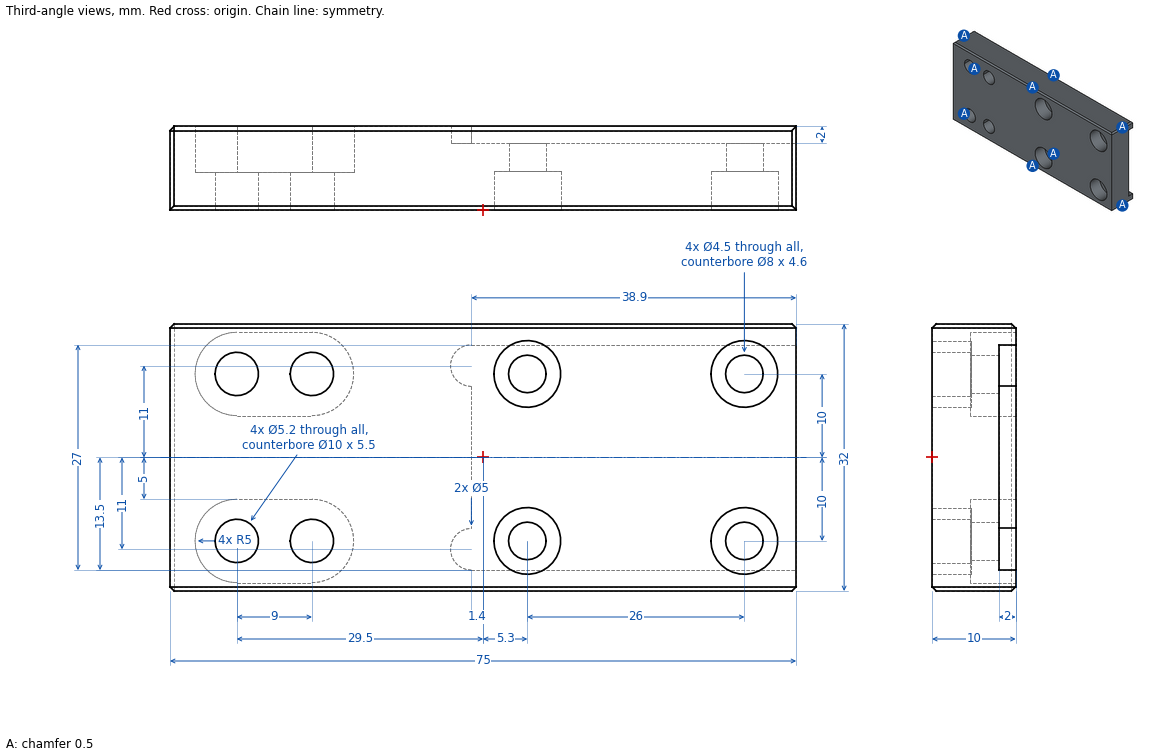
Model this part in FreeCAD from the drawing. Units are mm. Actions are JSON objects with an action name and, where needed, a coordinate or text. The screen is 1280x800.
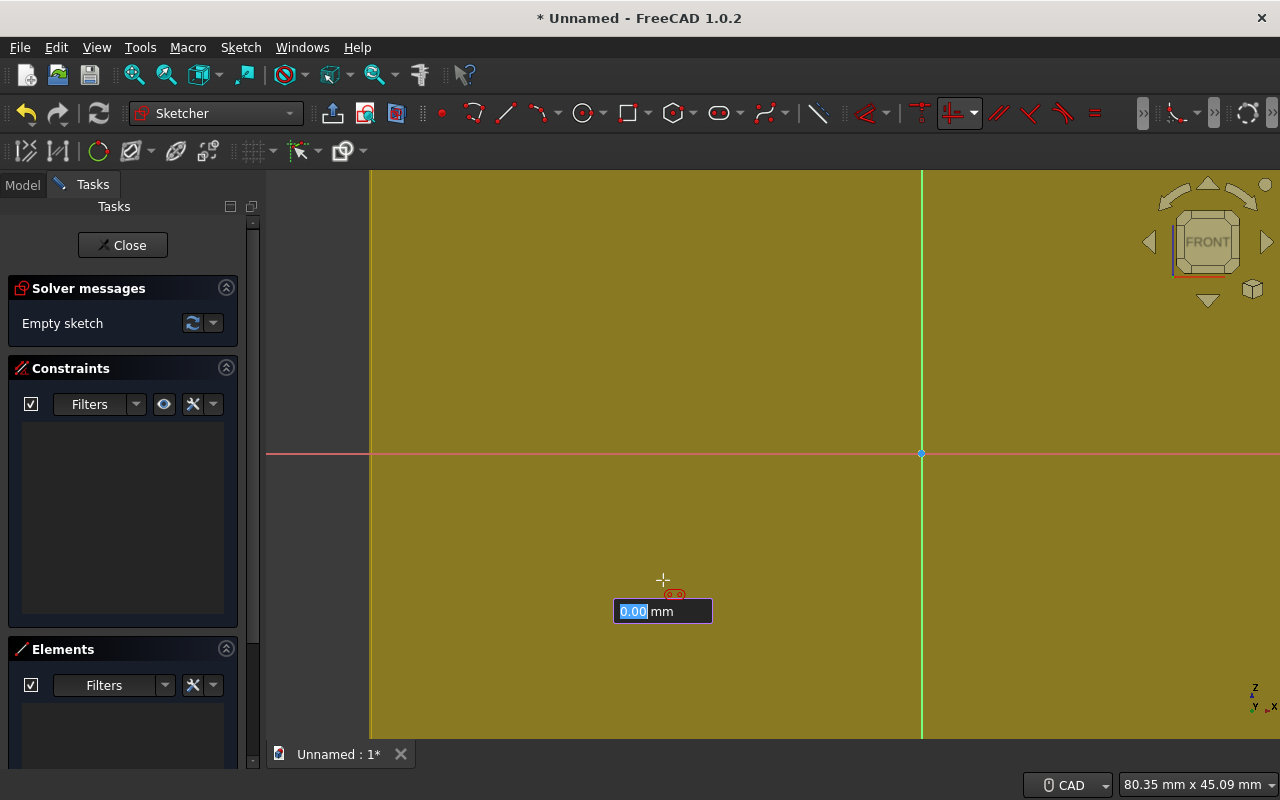
{"action": "left_click", "coordinate": [606, 643]}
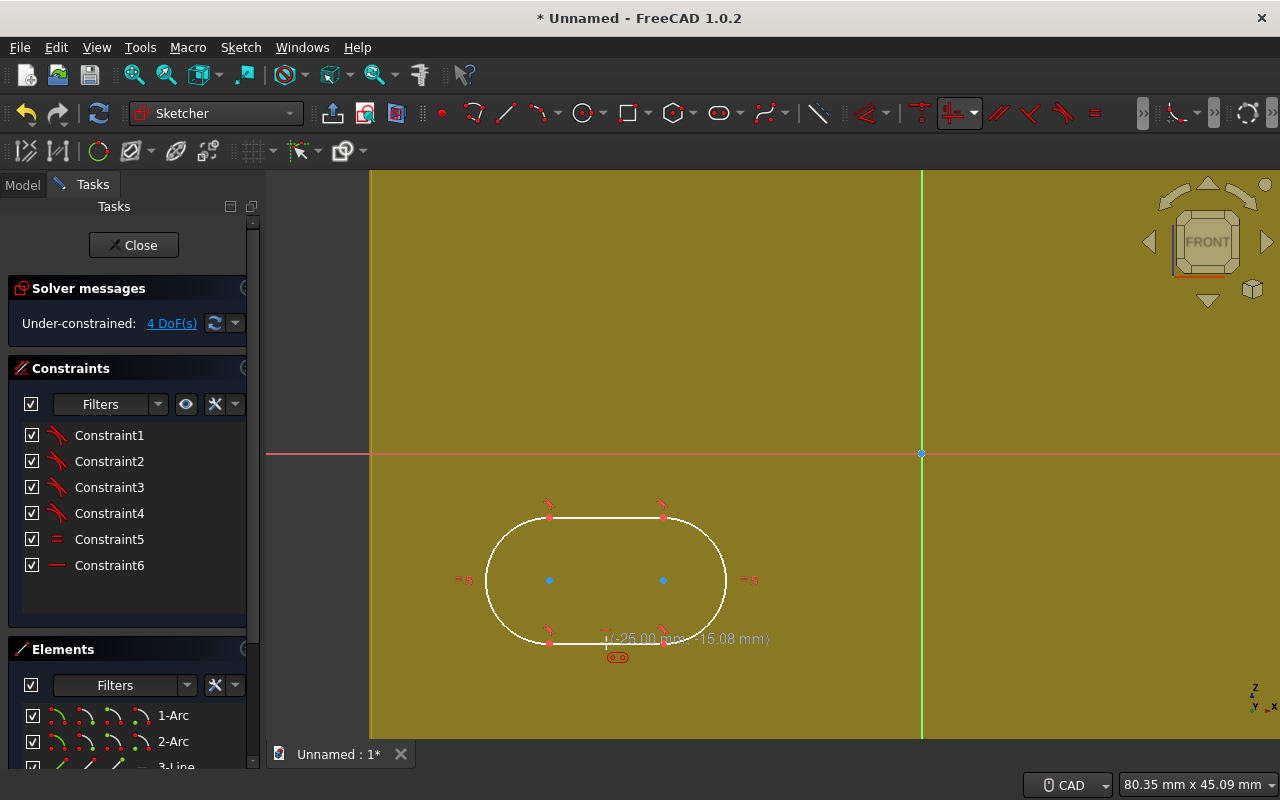
{"action": "left_click", "coordinate": [549, 327]}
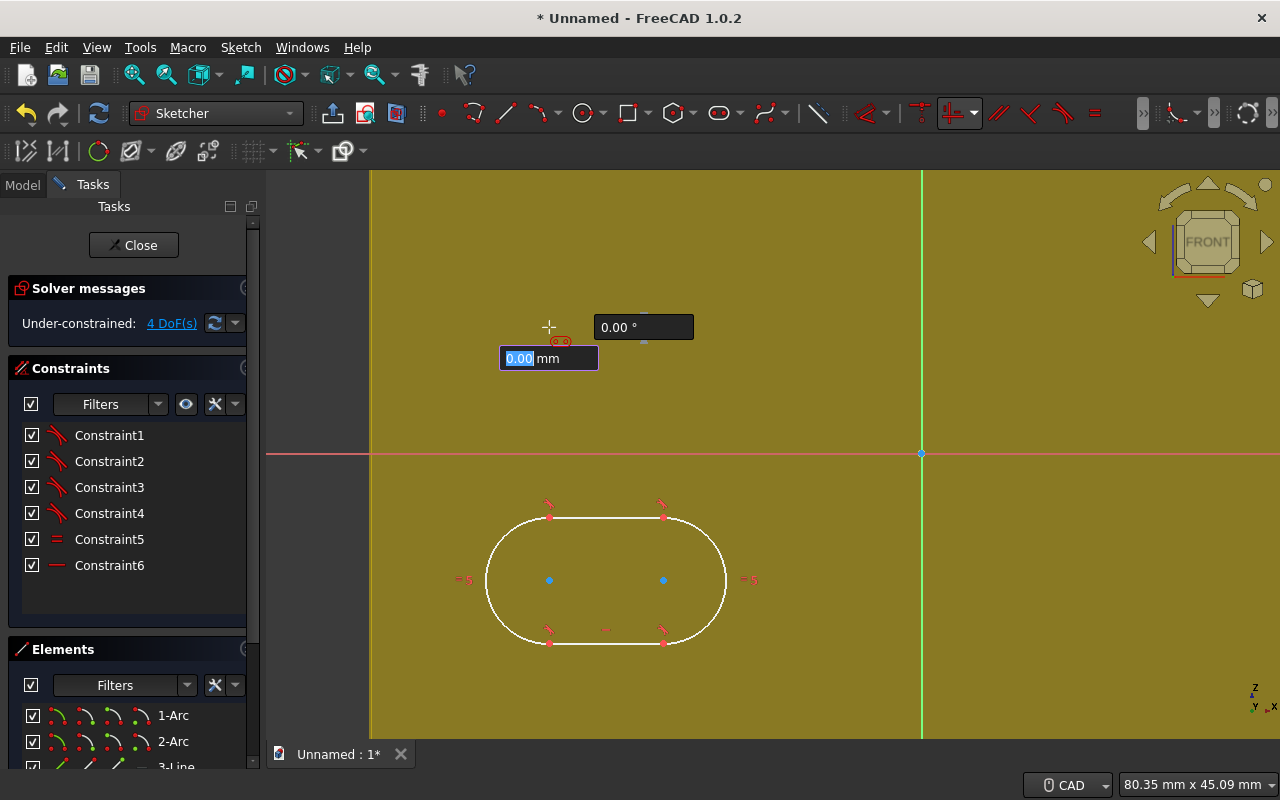
{"action": "left_click", "coordinate": [663, 327]}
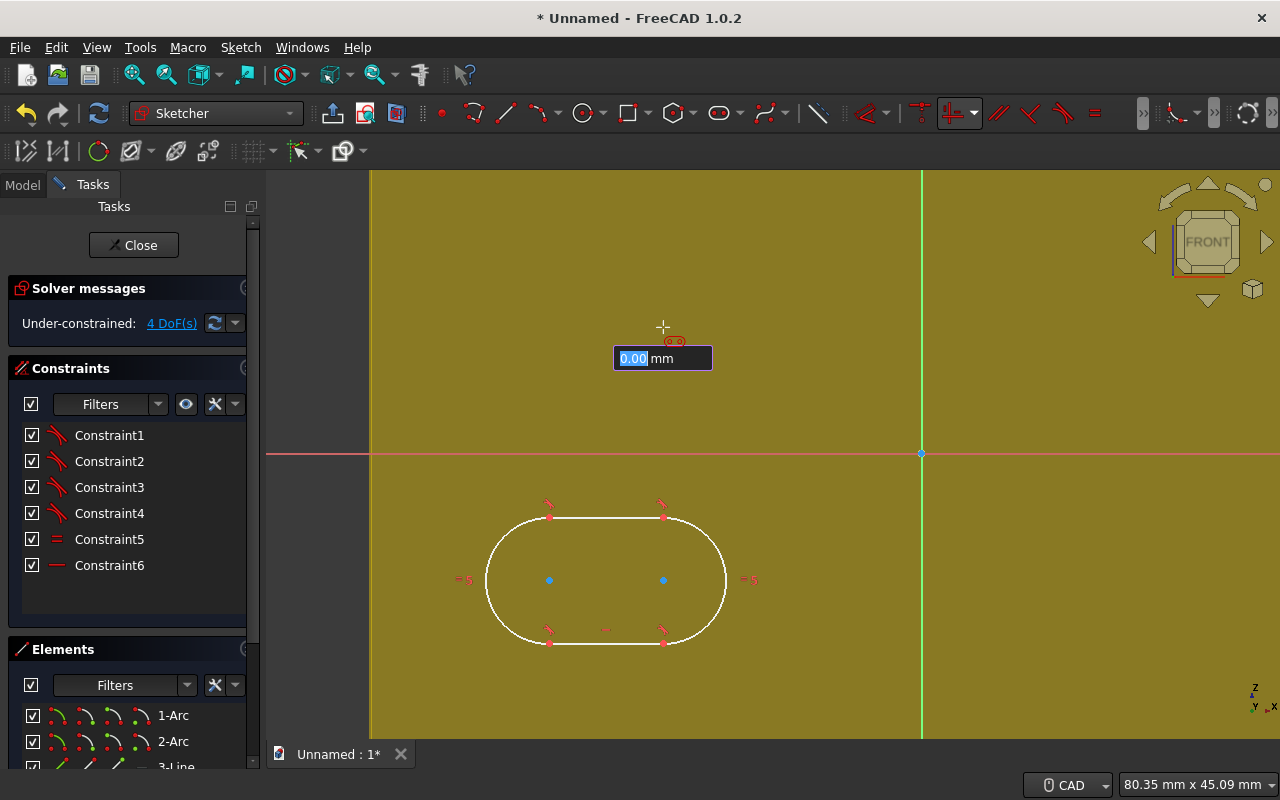
{"action": "left_click", "coordinate": [606, 391]}
{"action": "key", "text": "Escape"}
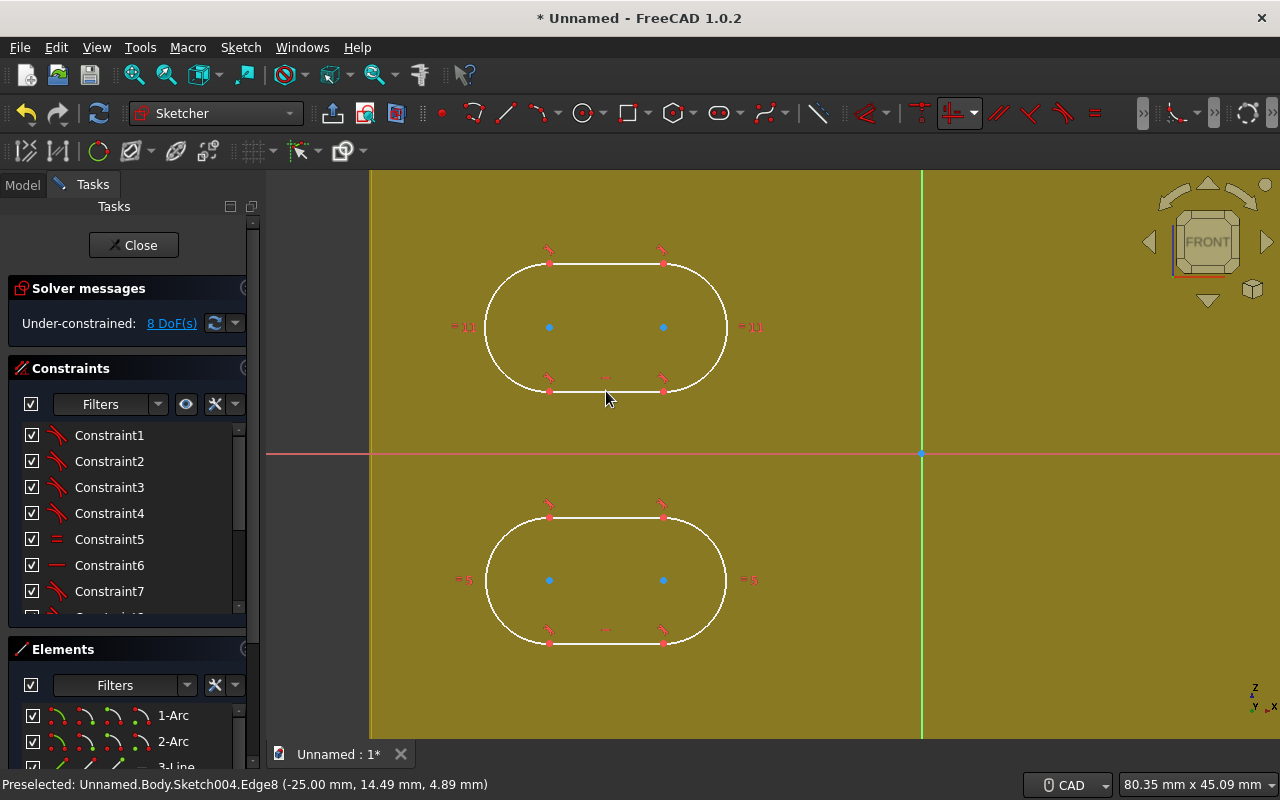
{"action": "left_click", "coordinate": [498, 544]}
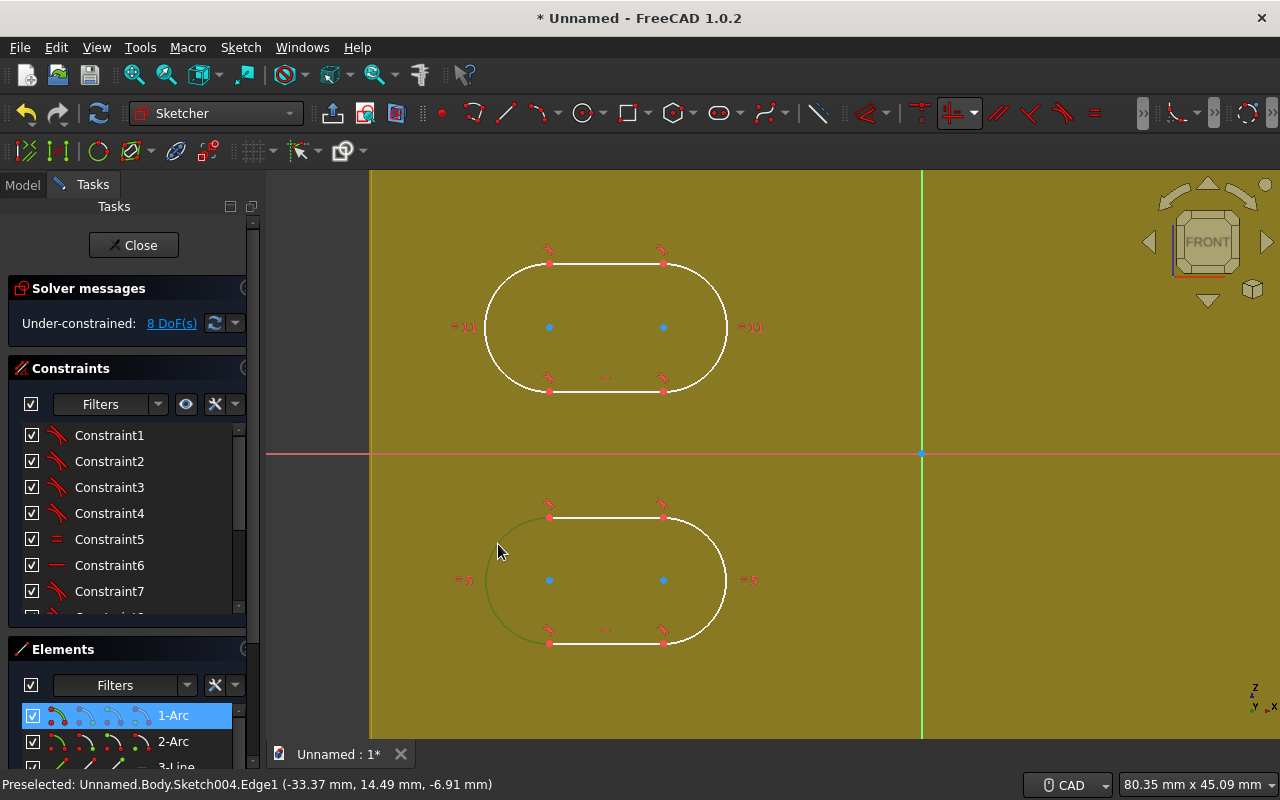
{"action": "left_click", "coordinate": [497, 290]}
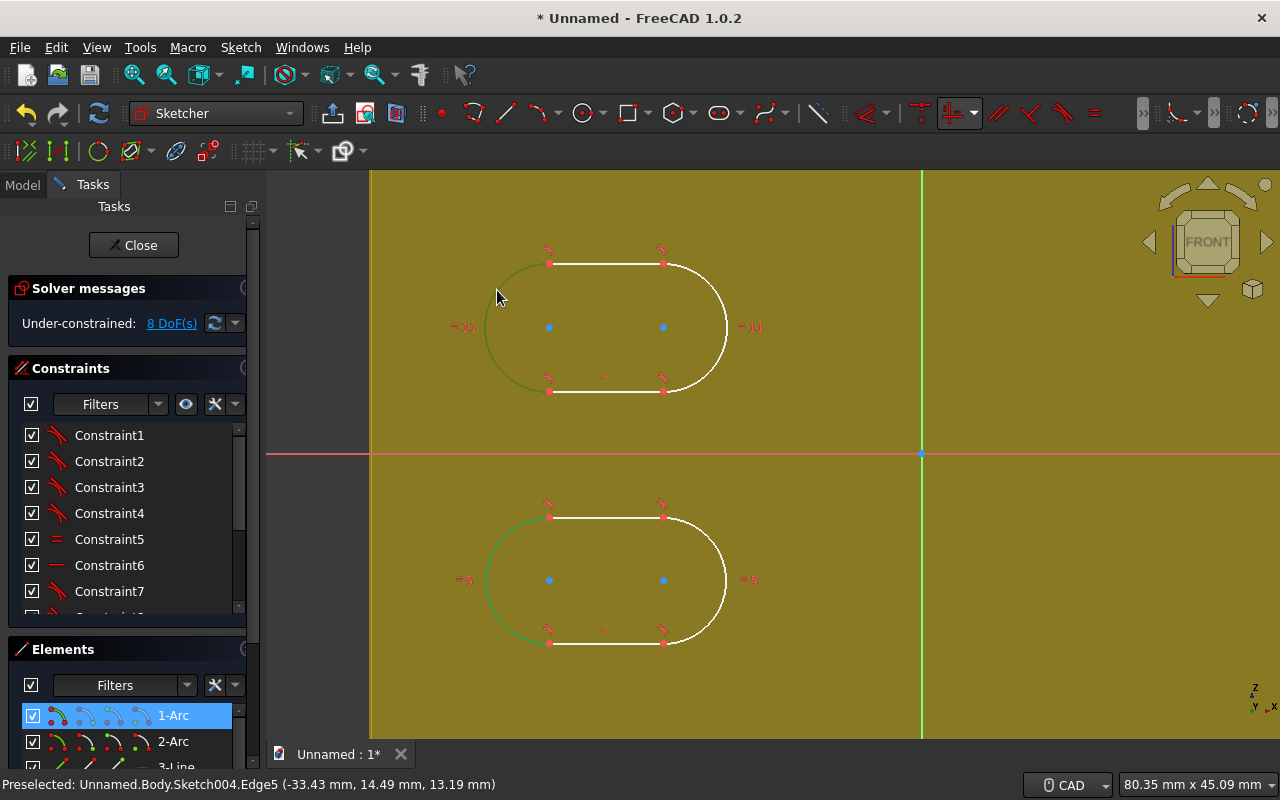
{"action": "left_click", "coordinate": [1096, 114]}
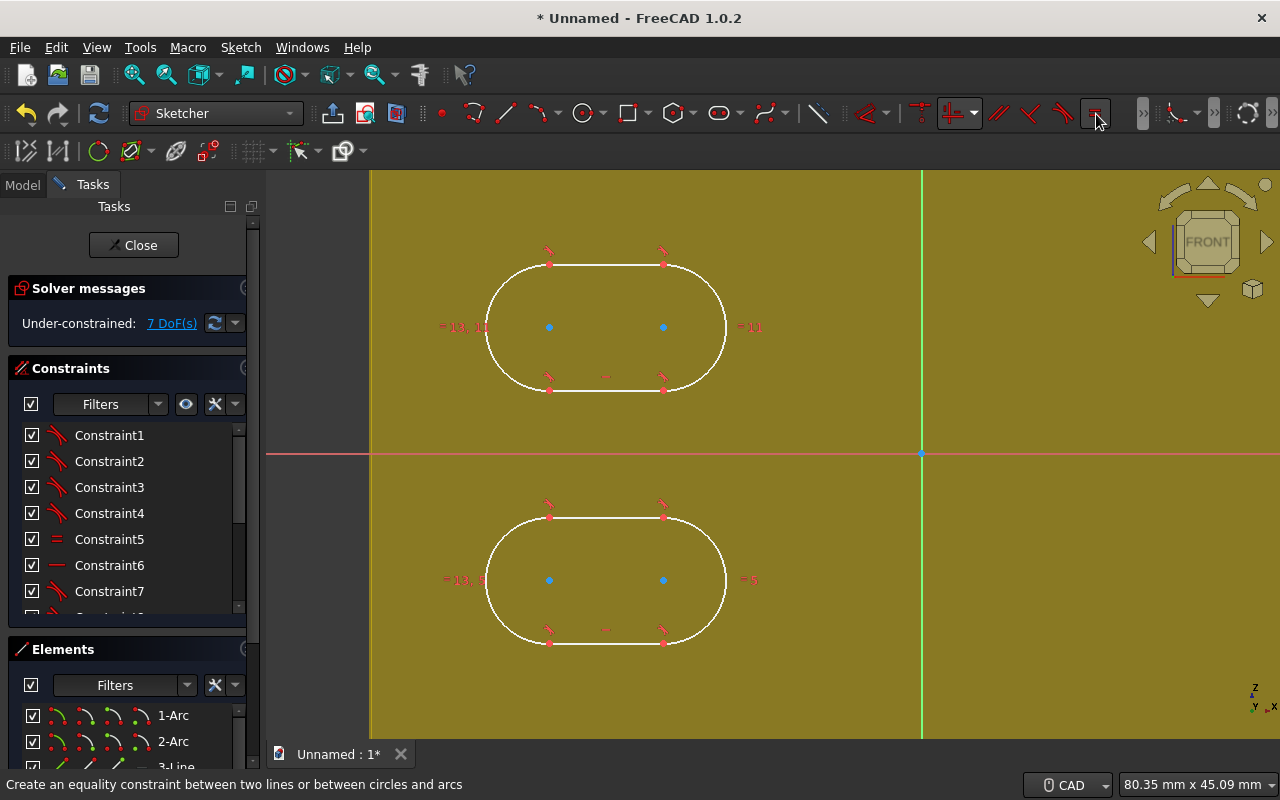
{"action": "left_click", "coordinate": [549, 581]}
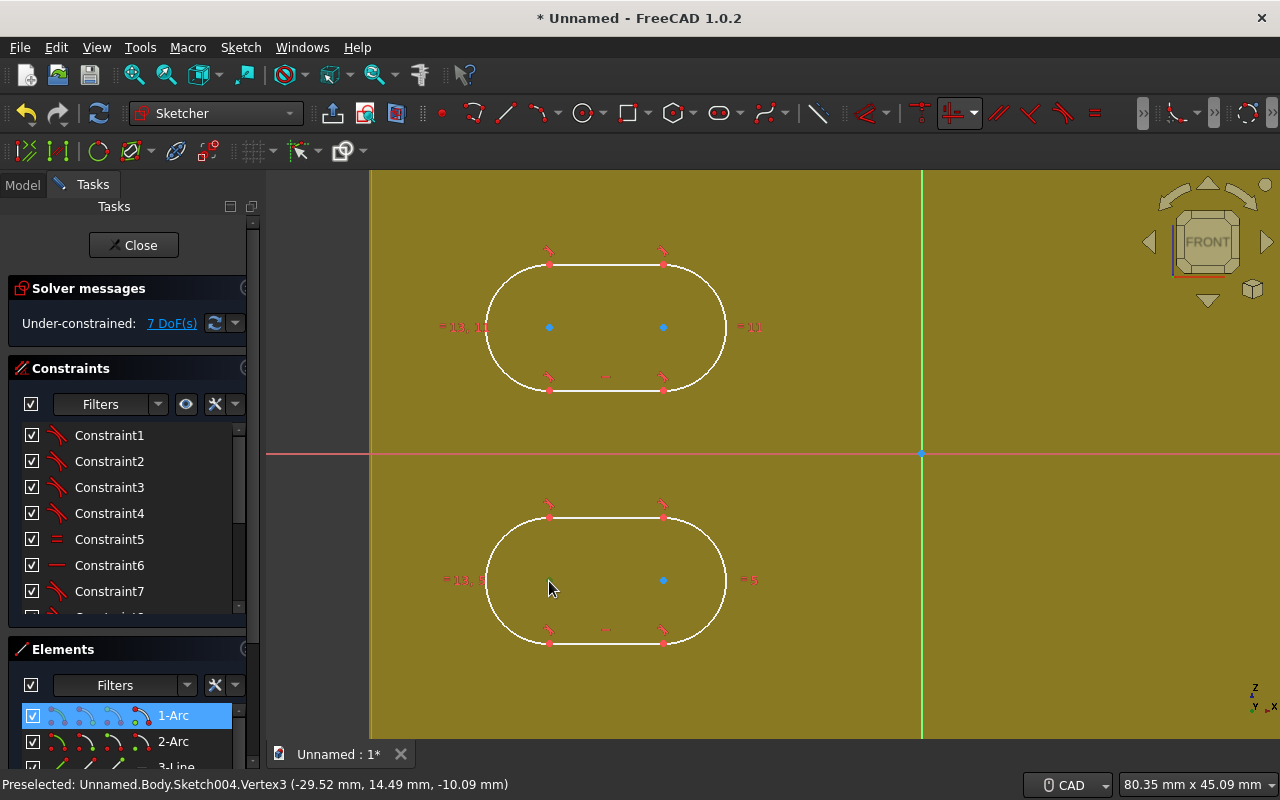
{"action": "left_click", "coordinate": [549, 328]}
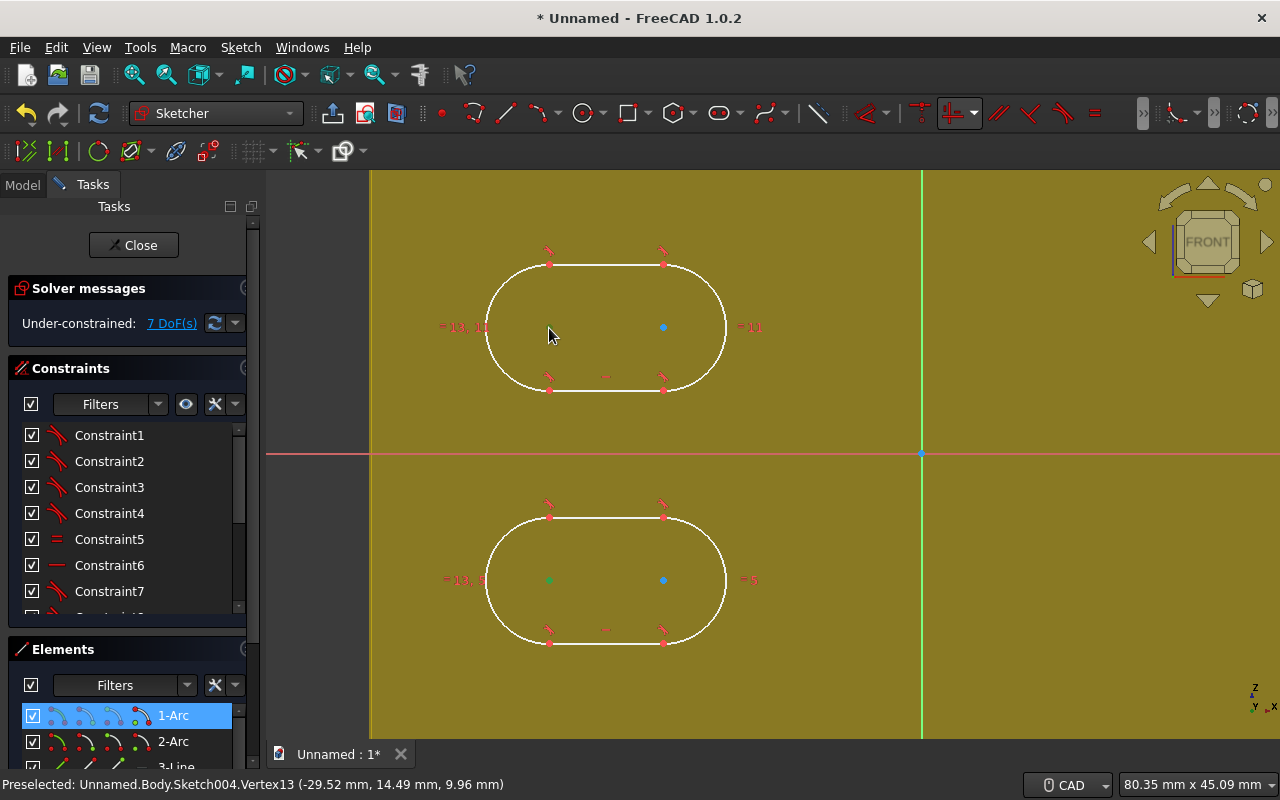
{"action": "left_click", "coordinate": [353, 454]}